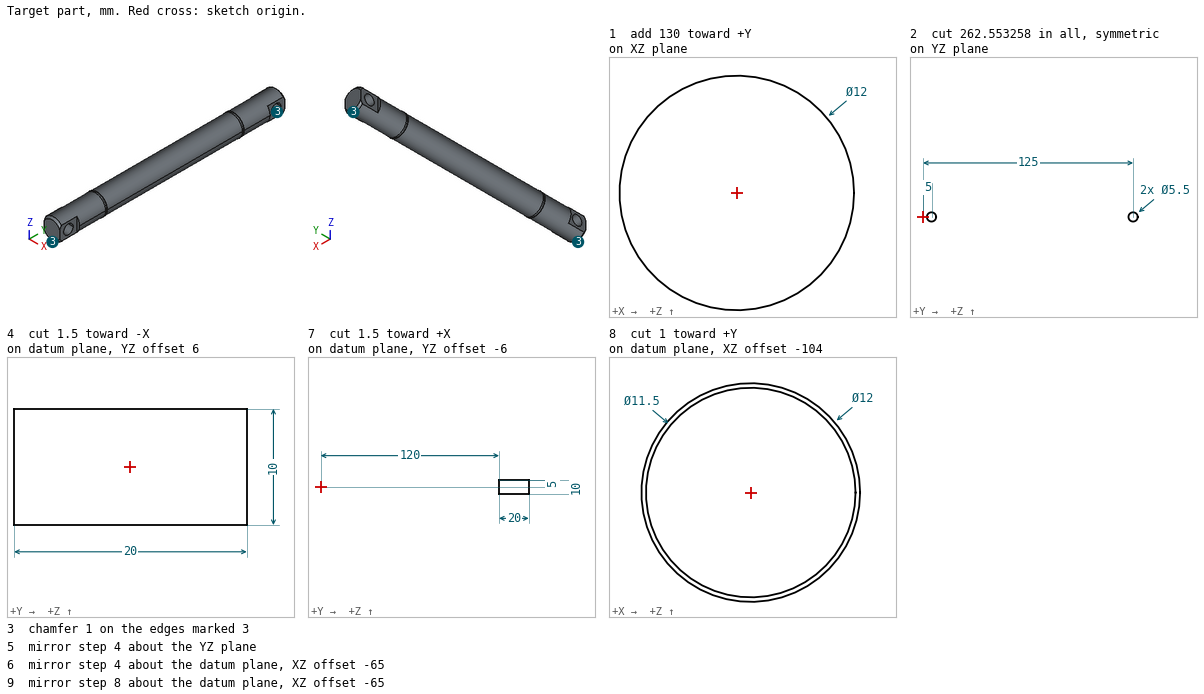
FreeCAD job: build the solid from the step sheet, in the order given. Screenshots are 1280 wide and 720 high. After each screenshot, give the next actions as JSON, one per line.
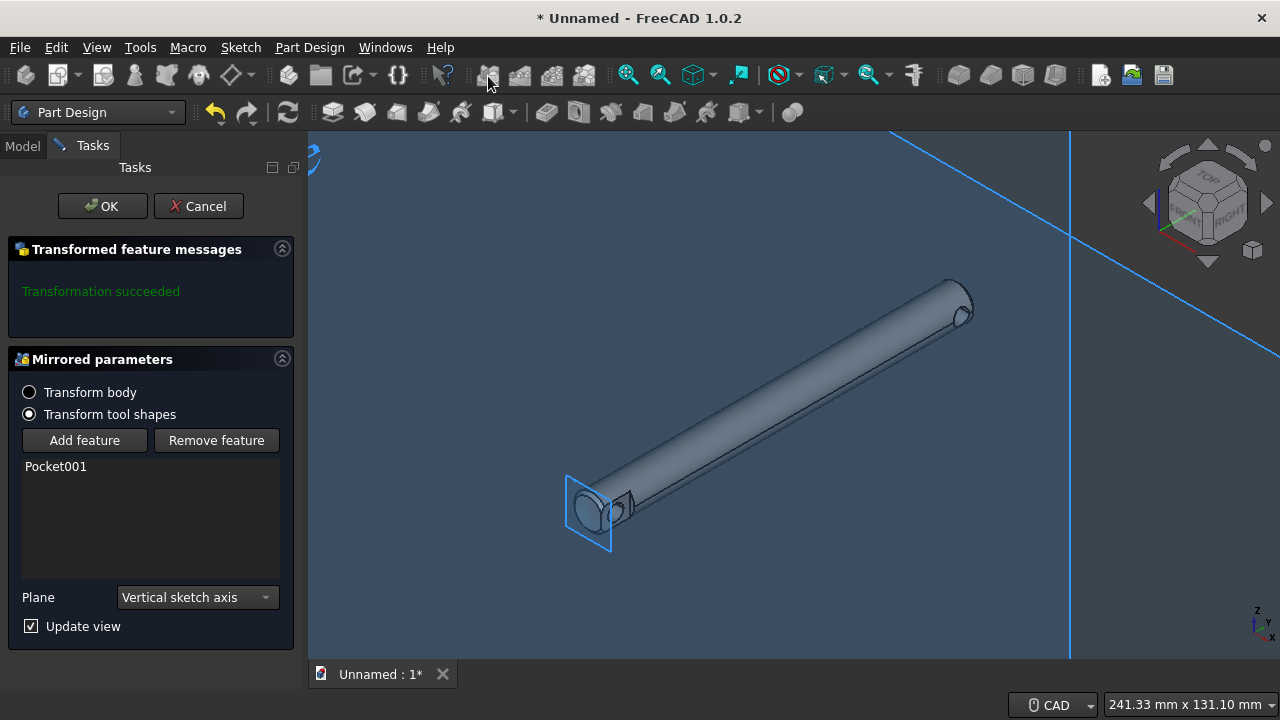
{"action": "left_click", "coordinate": [198, 598]}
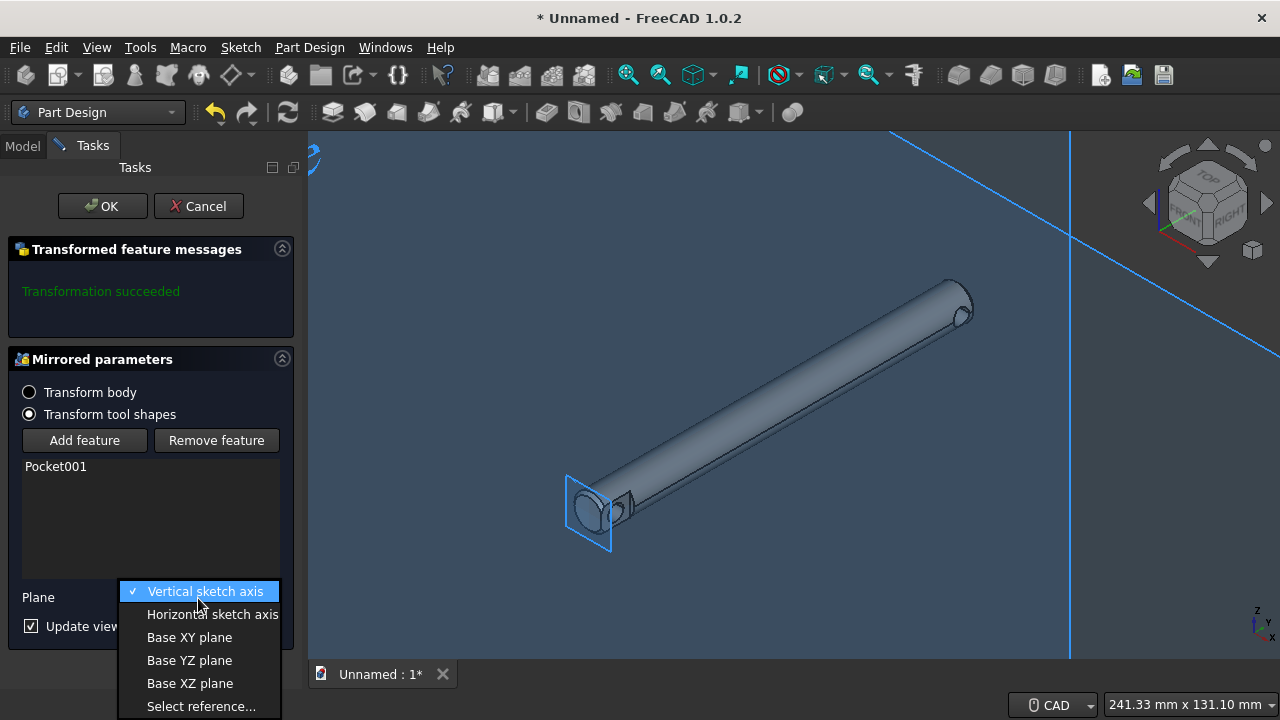
{"action": "left_click", "coordinate": [198, 660]}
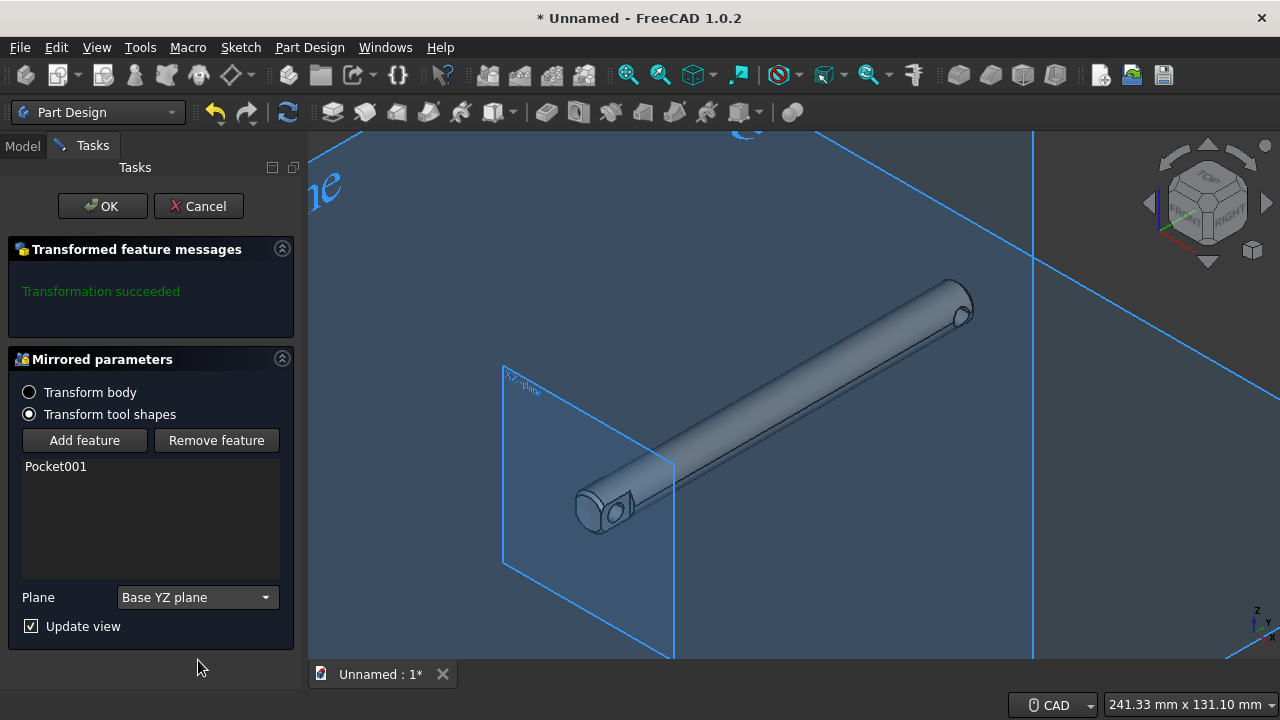
{"action": "left_click", "coordinate": [103, 206]}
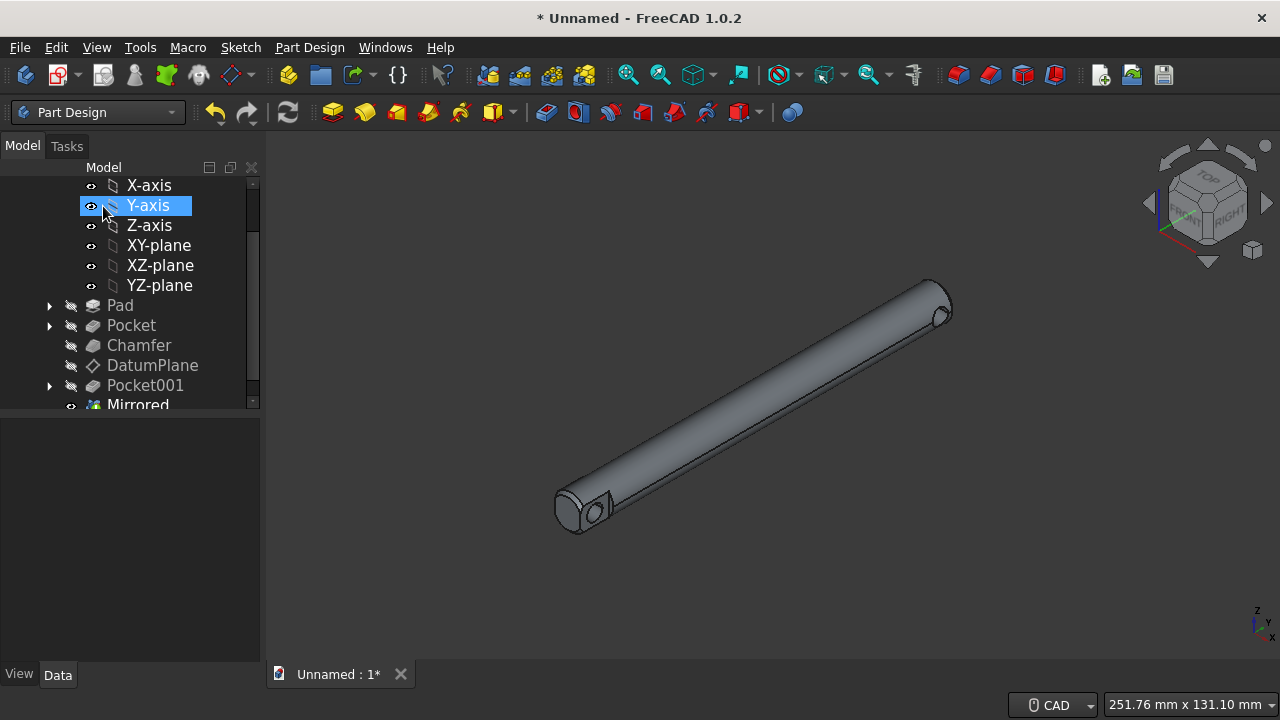
{"action": "scroll", "coordinate": [160, 301], "scroll_direction": "down", "scroll_amount": 3}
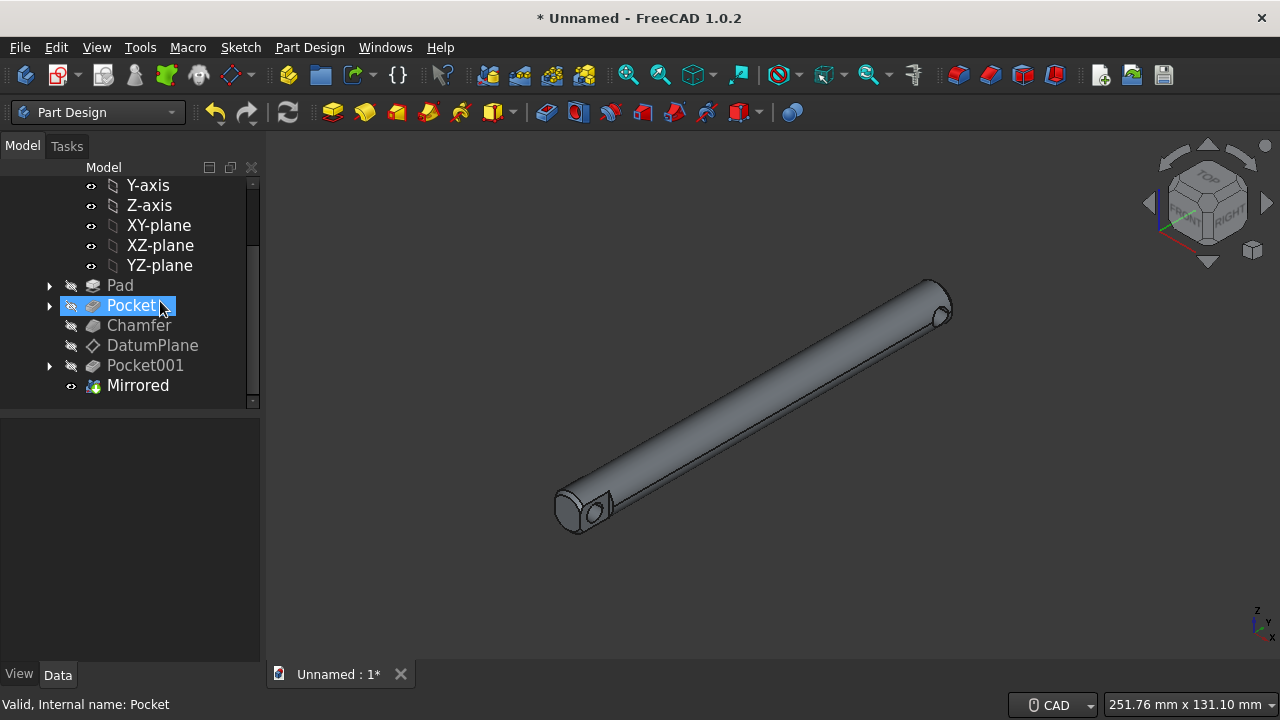
{"action": "scroll", "coordinate": [160, 281], "scroll_direction": "up", "scroll_amount": 15}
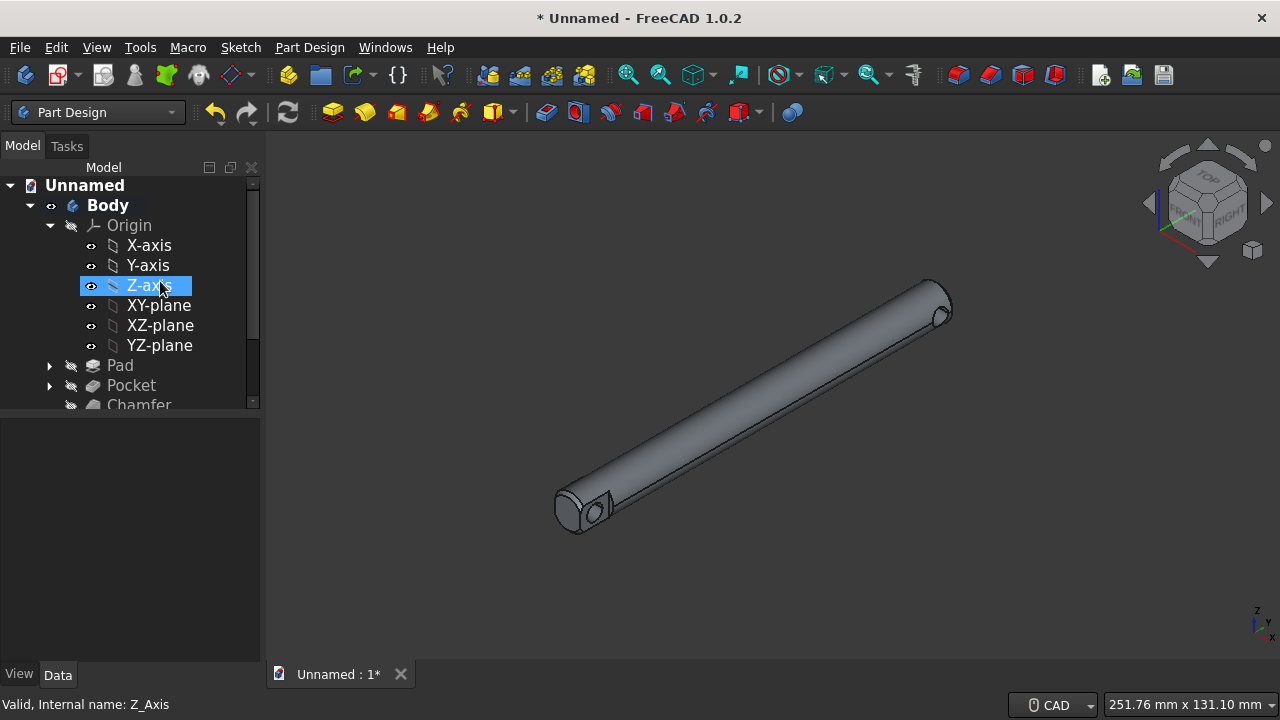
{"action": "left_click", "coordinate": [136, 326]}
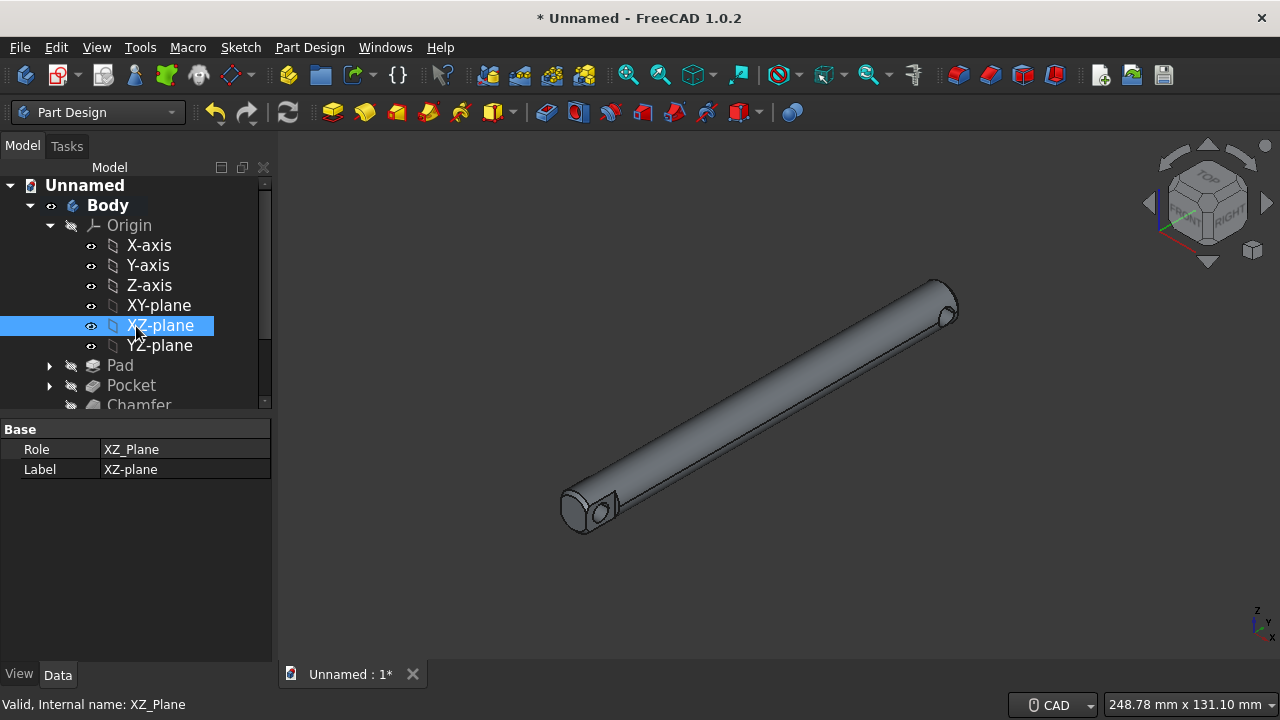
{"action": "left_click", "coordinate": [232, 76]}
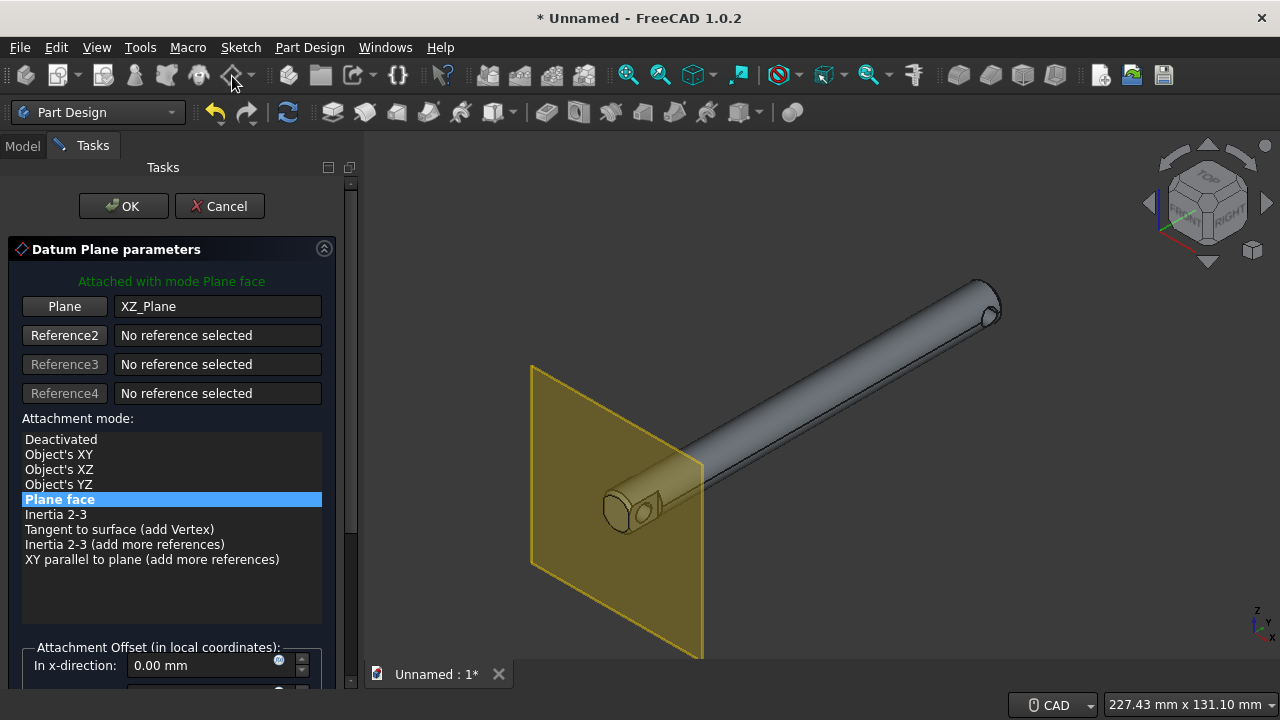
{"action": "scroll", "coordinate": [351, 432], "scroll_direction": "down", "scroll_amount": 2}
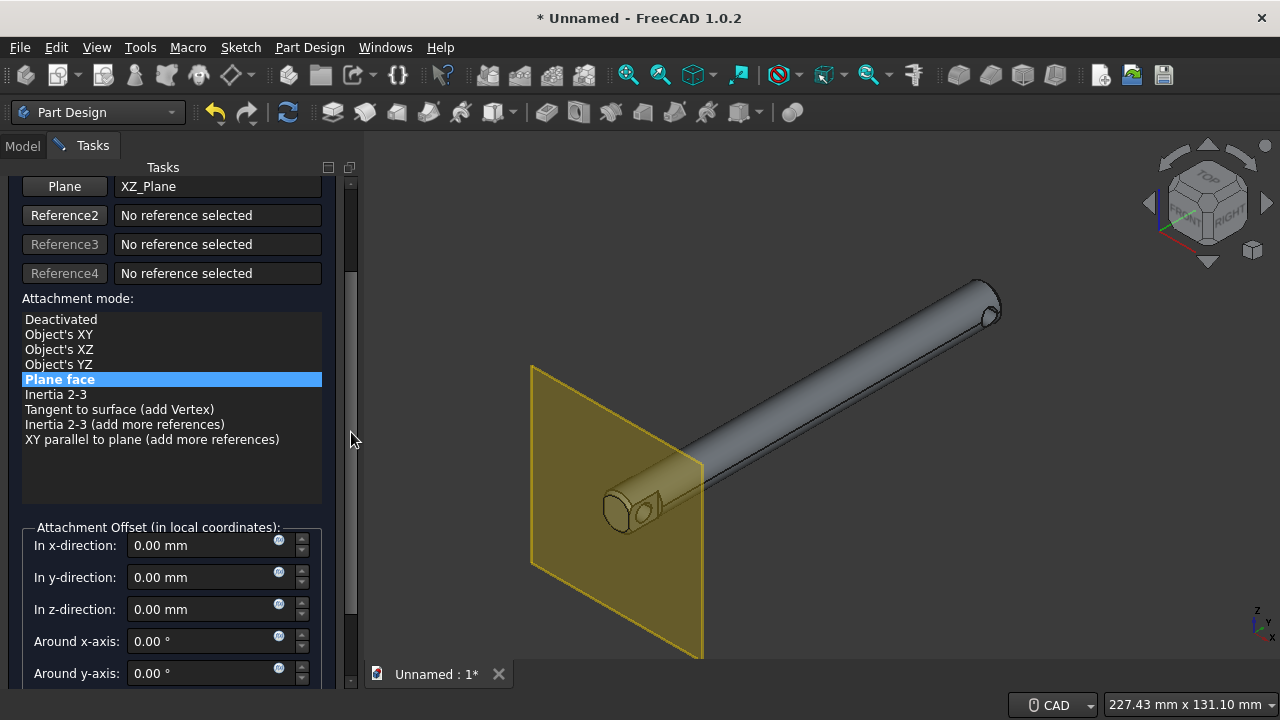
{"action": "triple_click", "coordinate": [210, 609]}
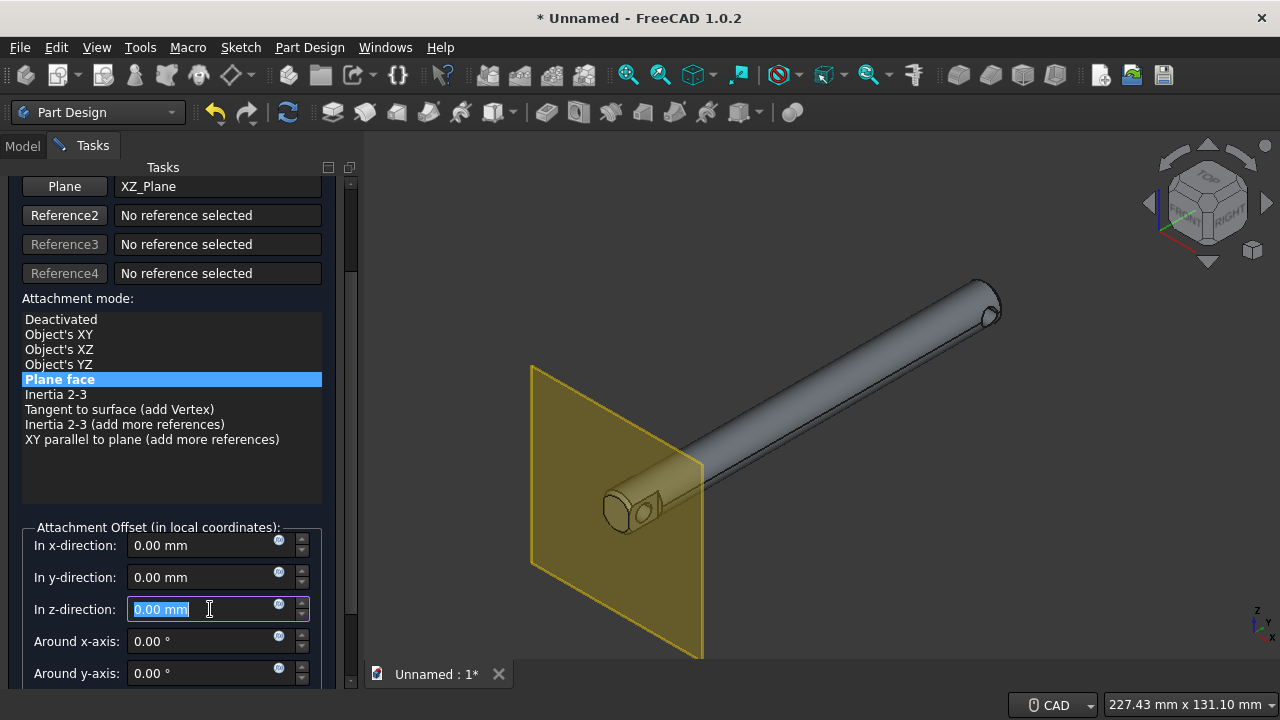
{"action": "type", "text": "-65"}
{"action": "key", "text": "Tab"}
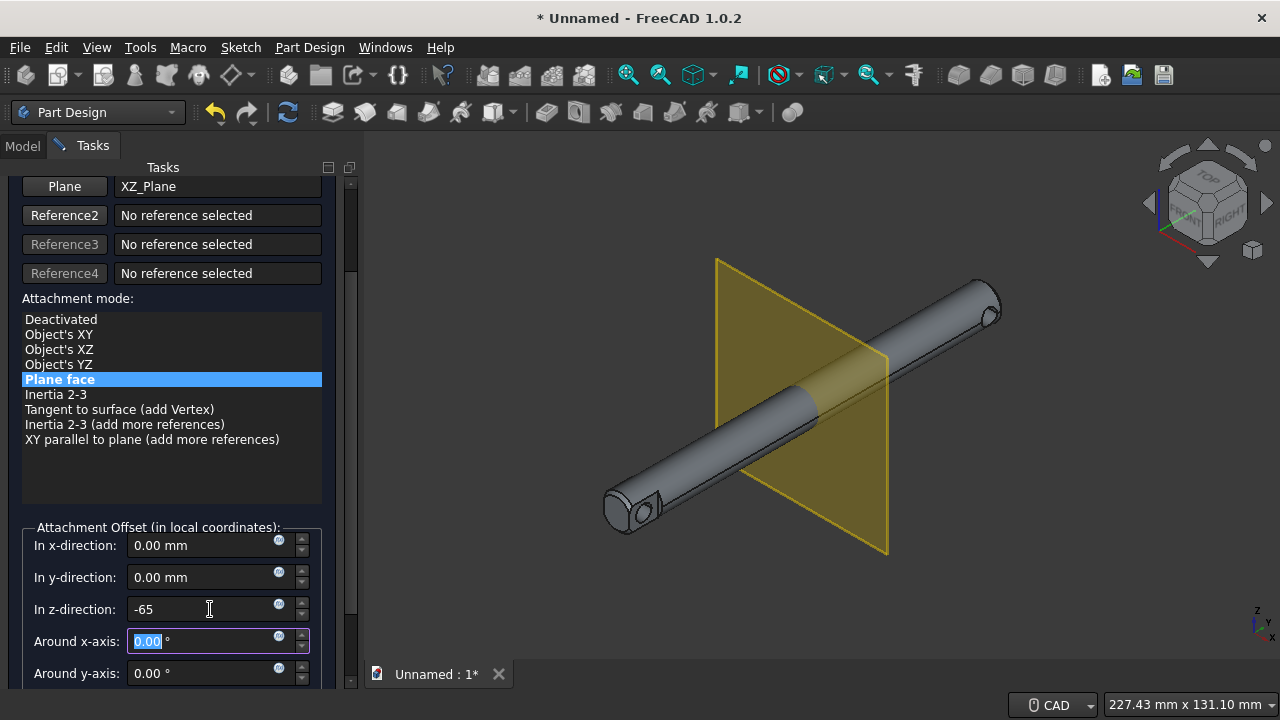
{"action": "scroll", "coordinate": [351, 432], "scroll_direction": "up", "scroll_amount": 3}